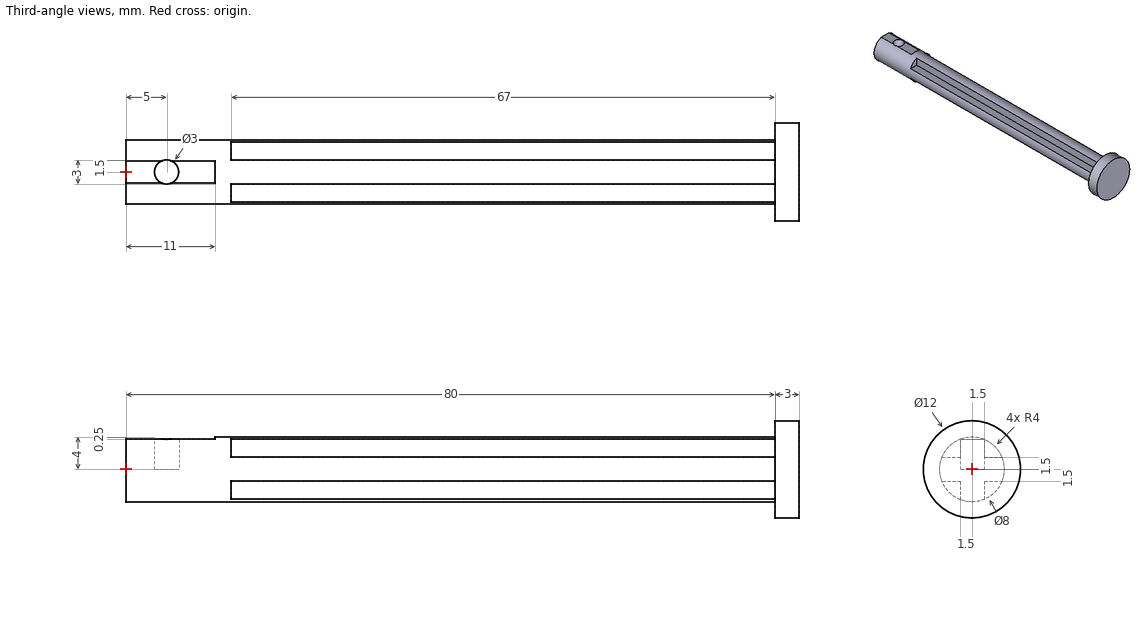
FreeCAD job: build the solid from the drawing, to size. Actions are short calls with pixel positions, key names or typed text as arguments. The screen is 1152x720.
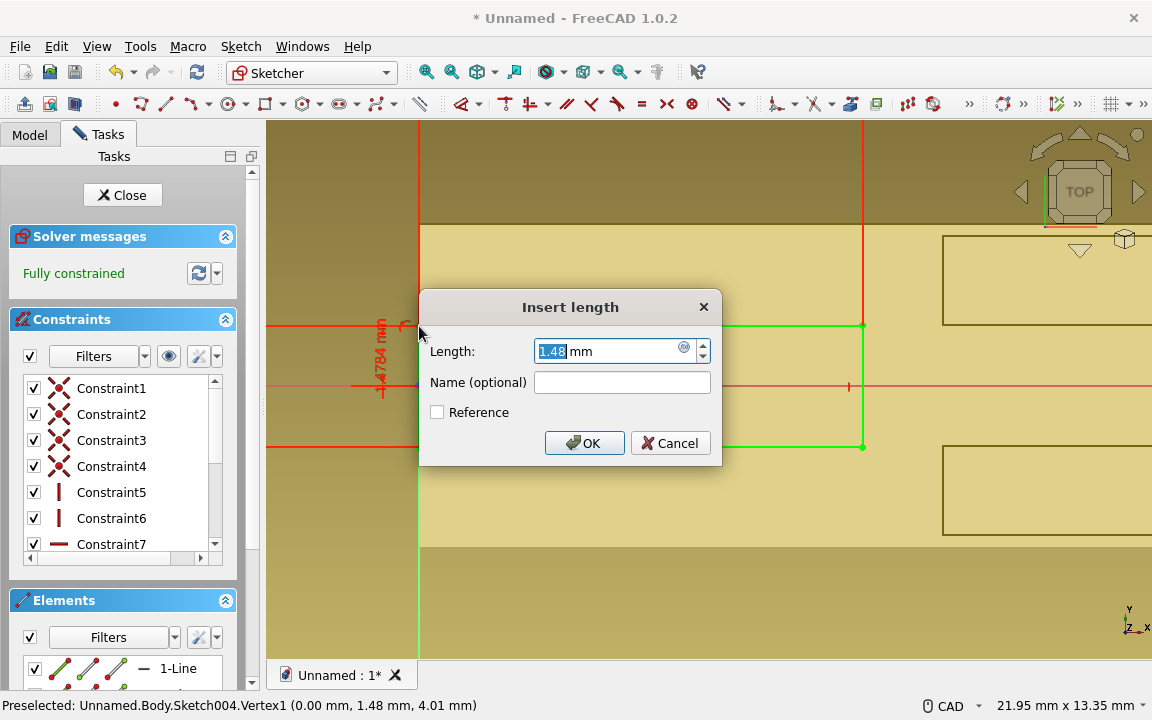
text(1.5)
key(Return)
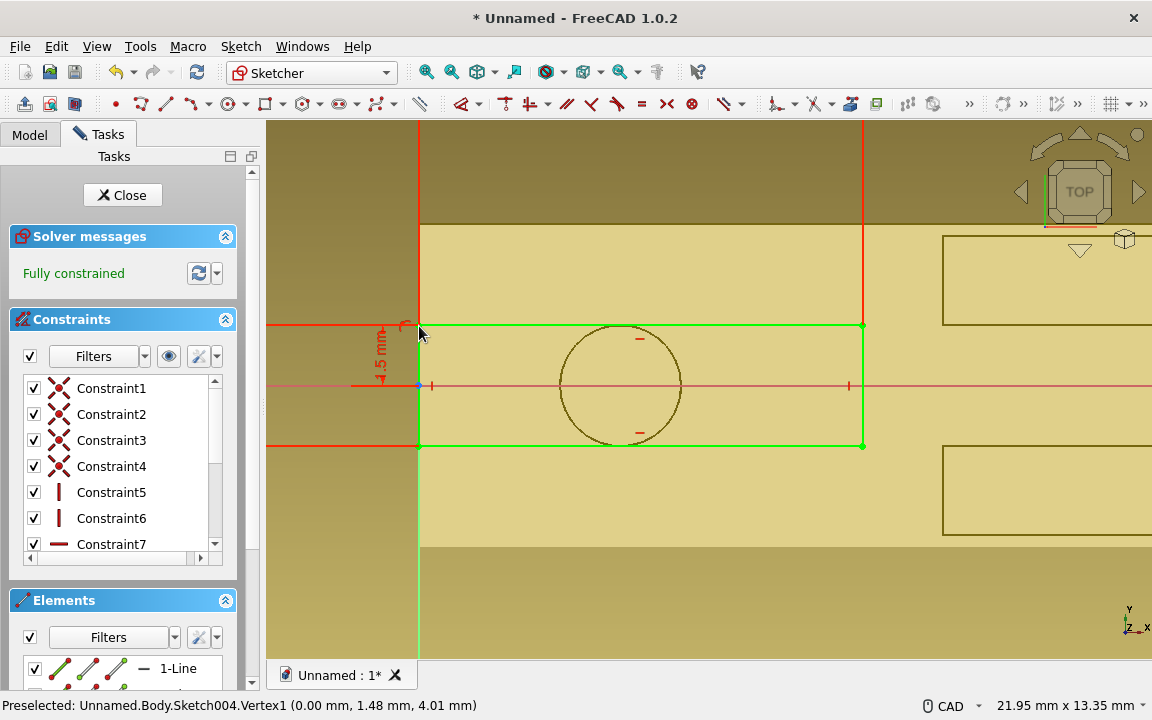
click(123, 195)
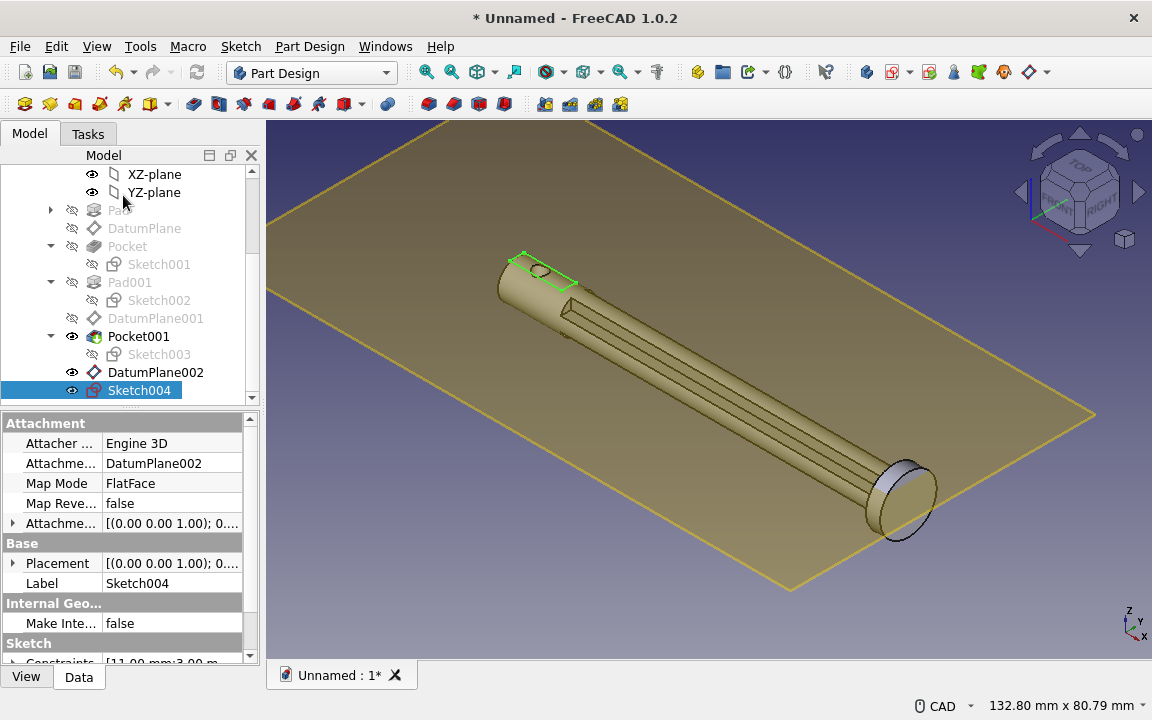
click(194, 104)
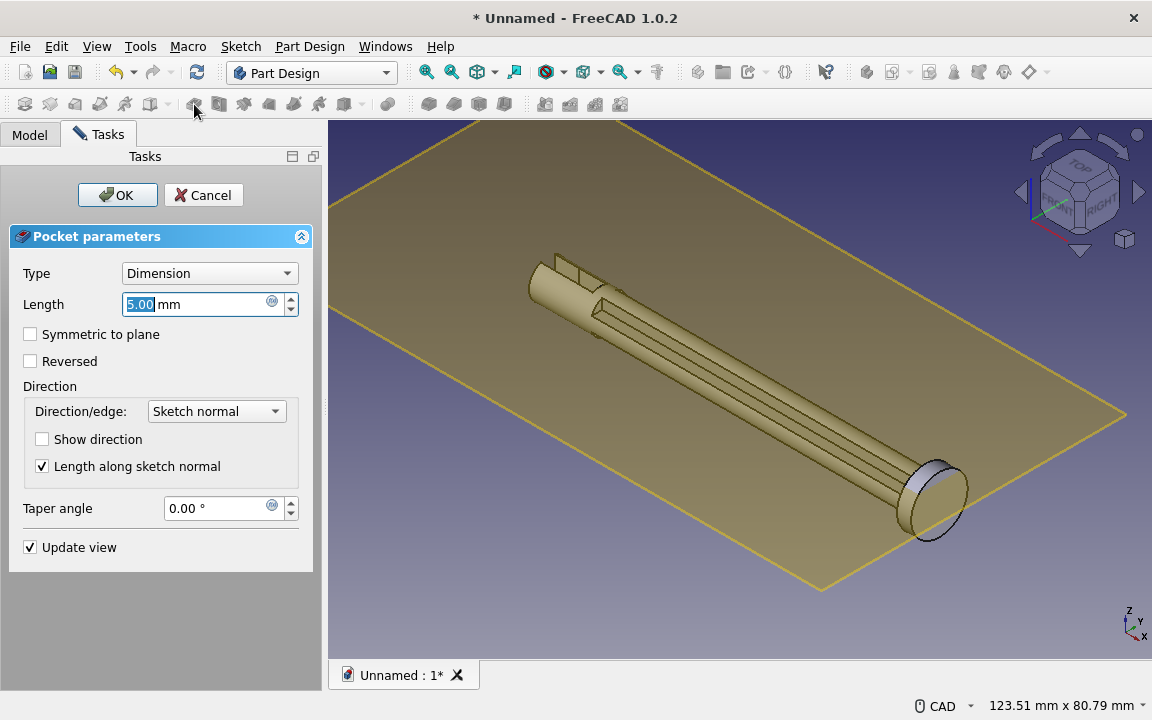
text(0.25)
key(Tab)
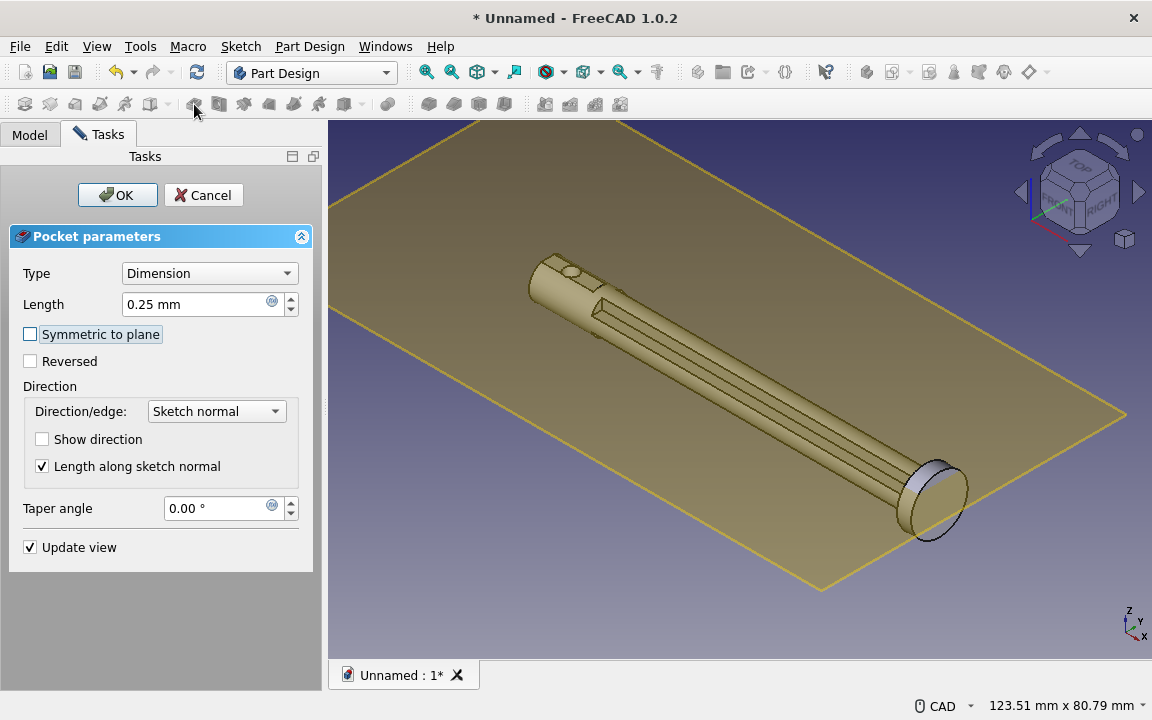
click(118, 195)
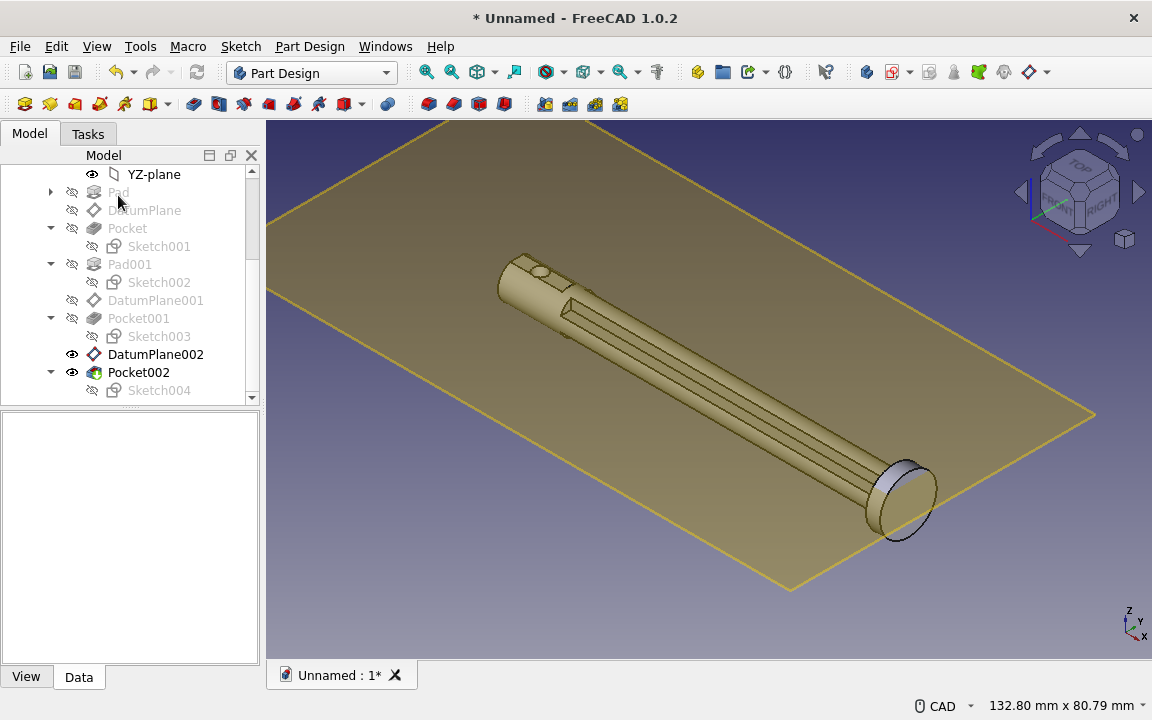
click(117, 354)
key(space)